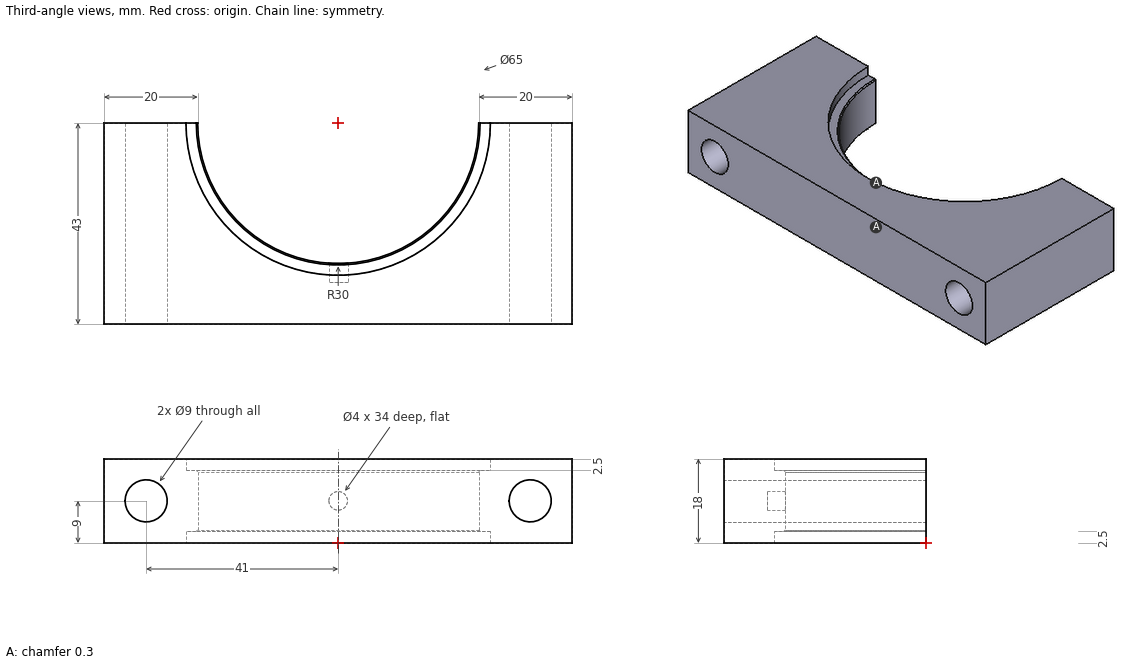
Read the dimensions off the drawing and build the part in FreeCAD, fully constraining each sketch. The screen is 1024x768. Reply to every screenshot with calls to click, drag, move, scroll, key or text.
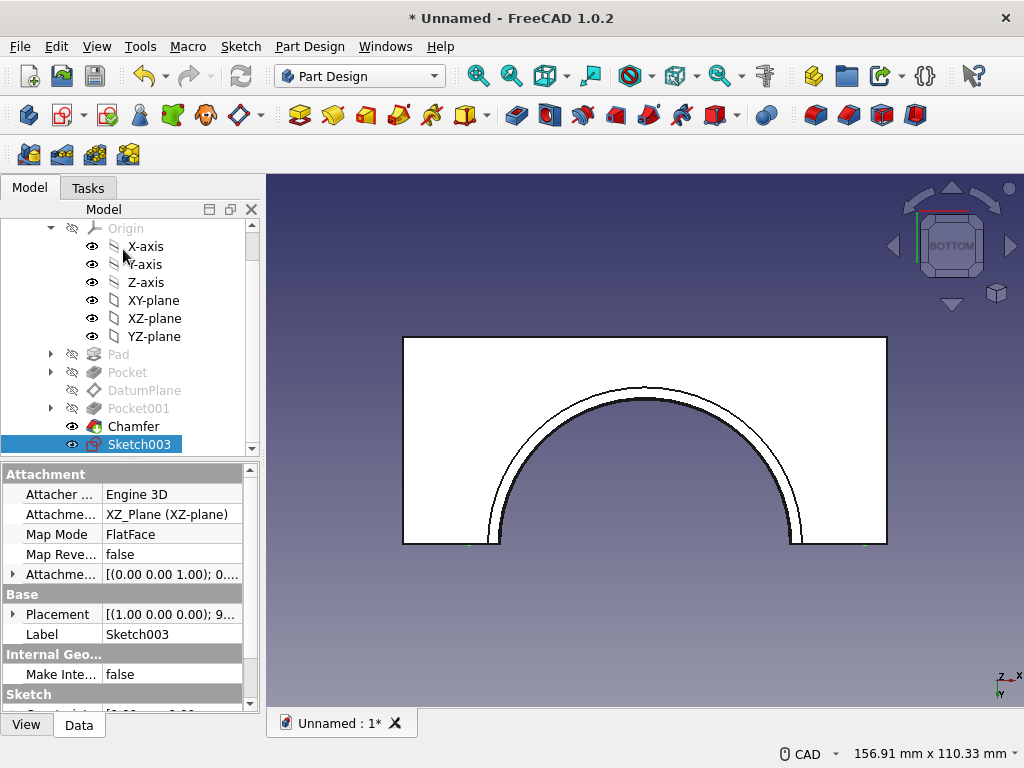
click(550, 116)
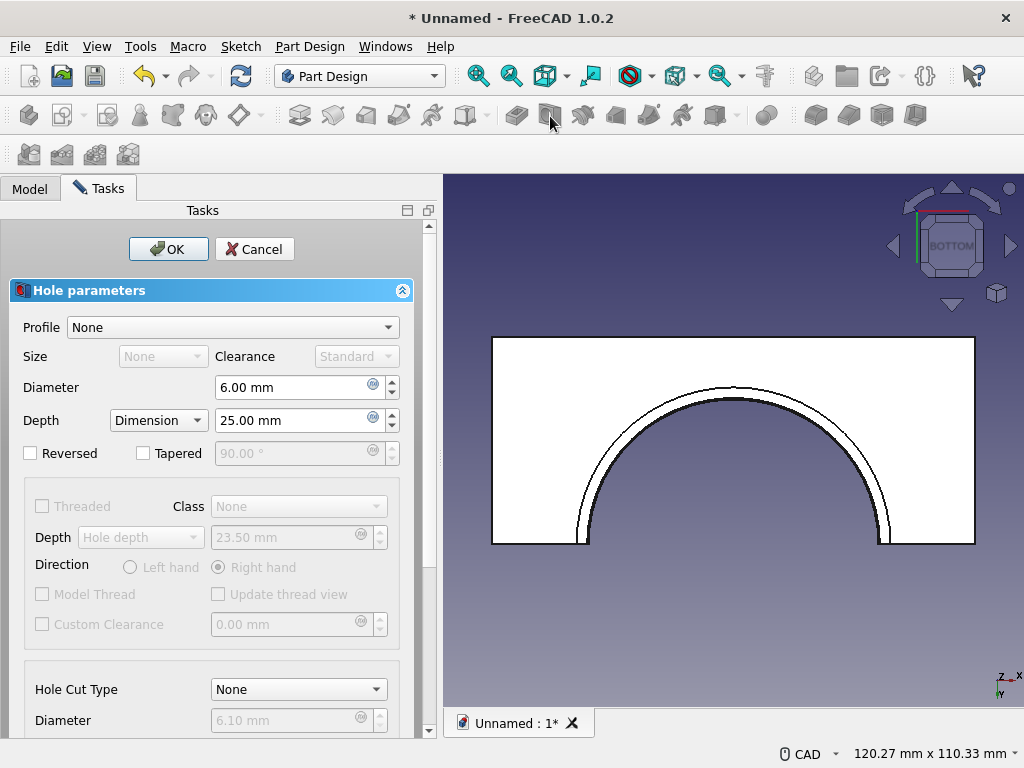
triple_click(300, 388)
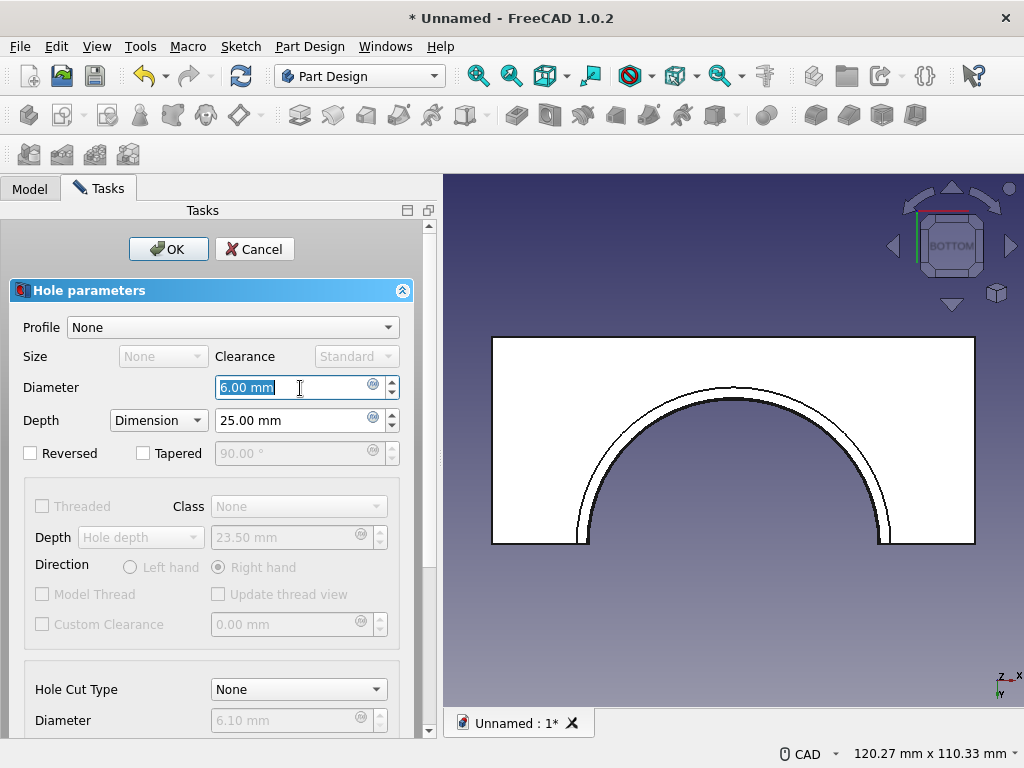
text(9)
key(Tab)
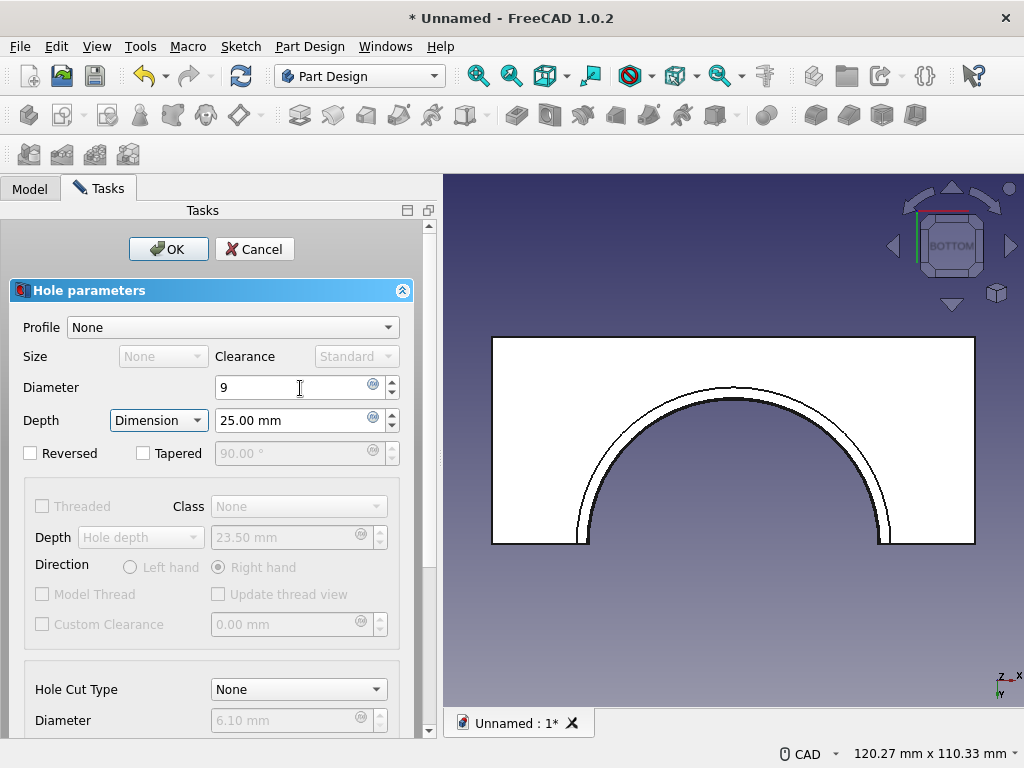
click(160, 420)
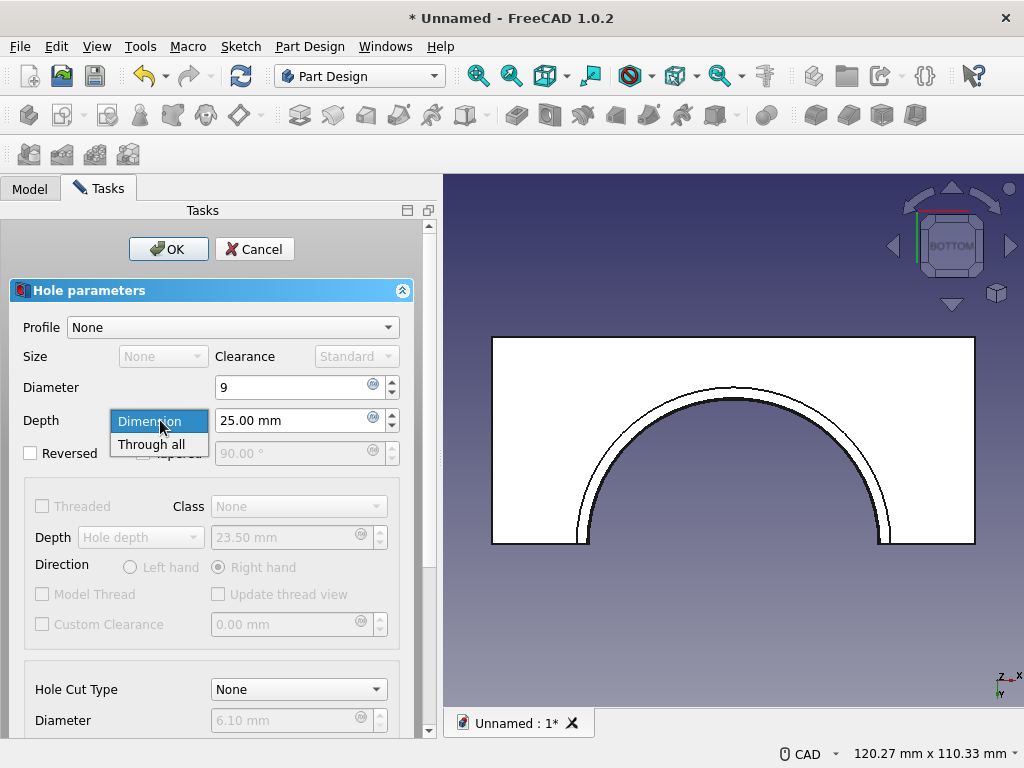
click(158, 444)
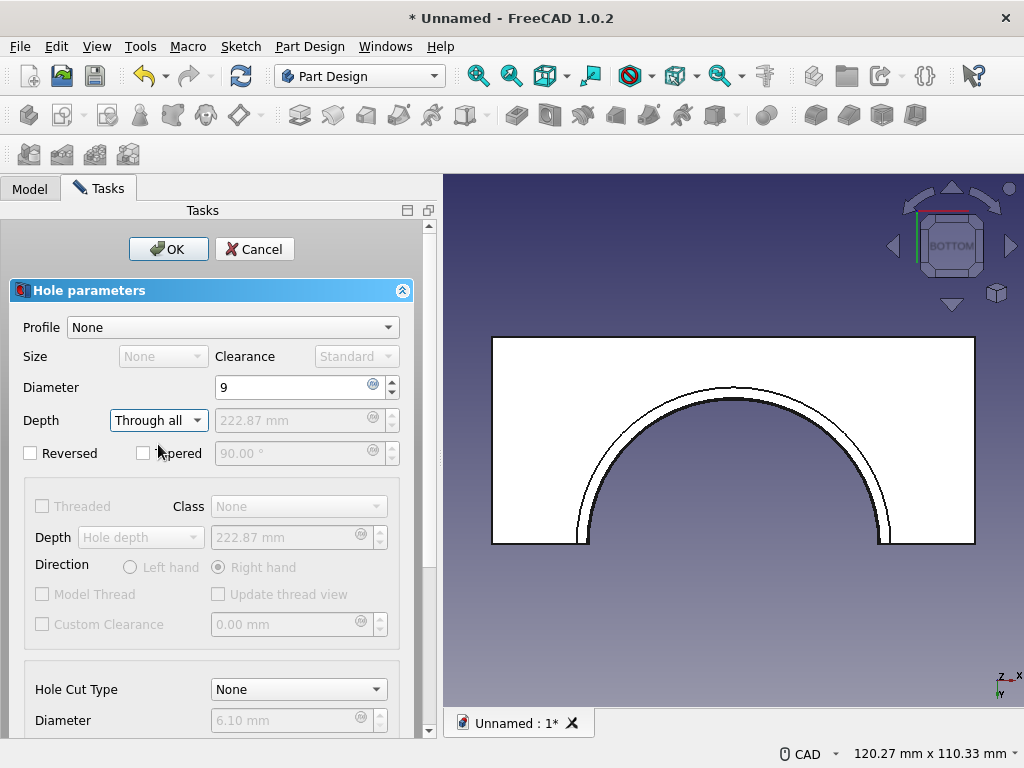
click(31, 453)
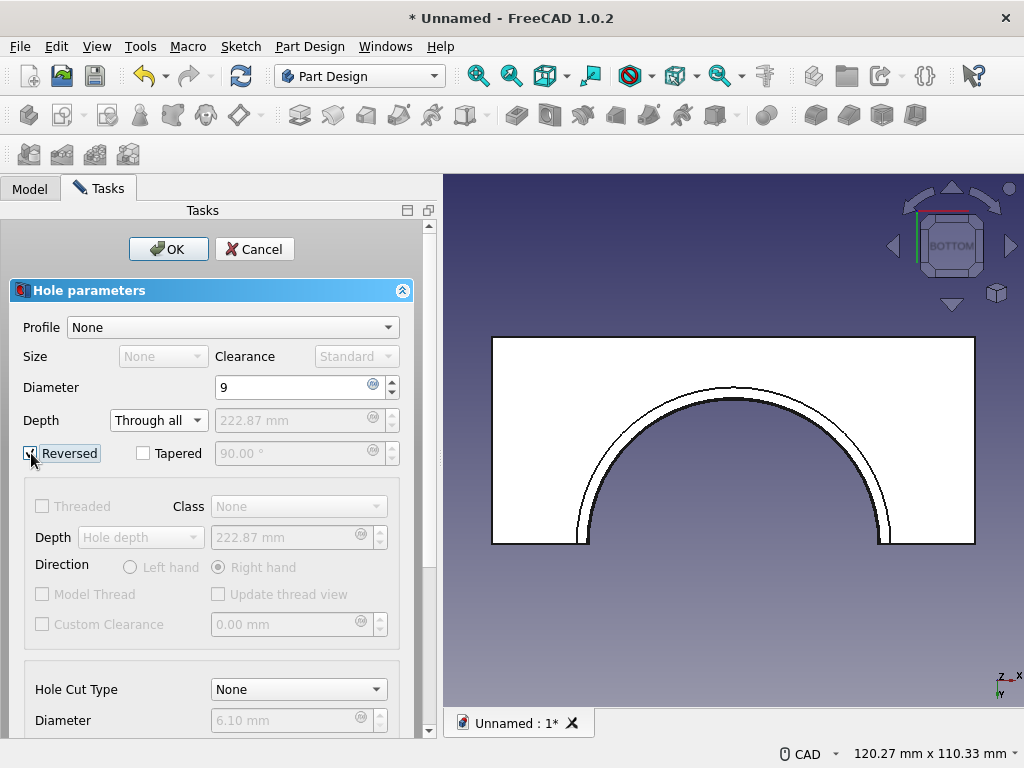
click(169, 249)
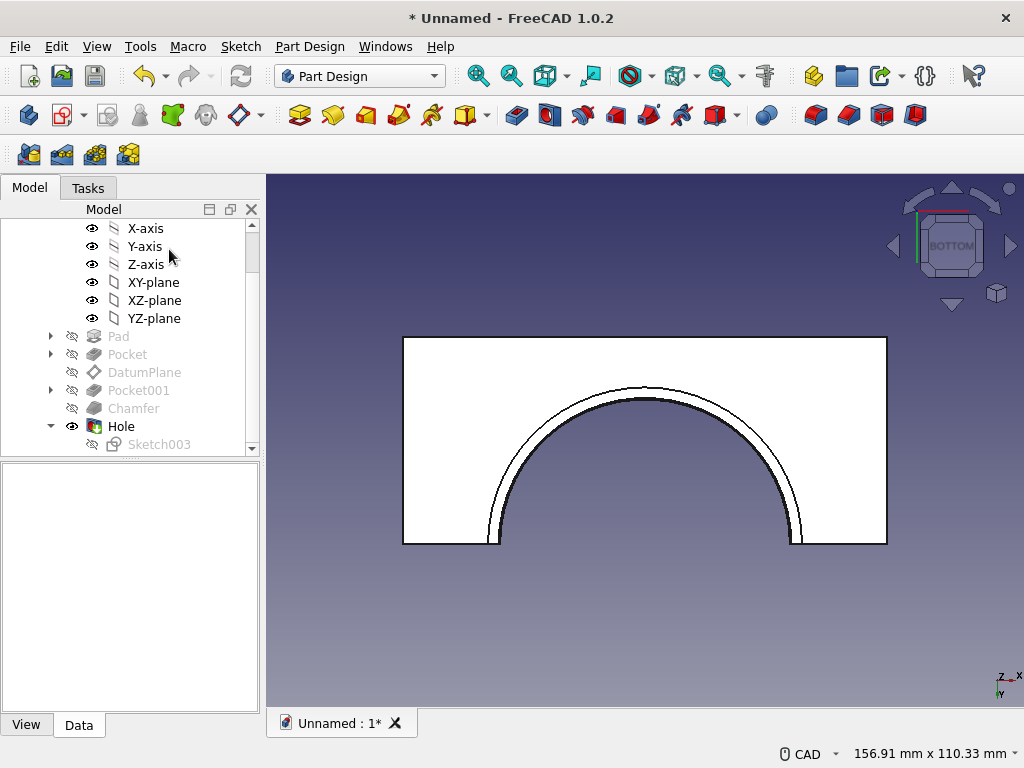
click(62, 116)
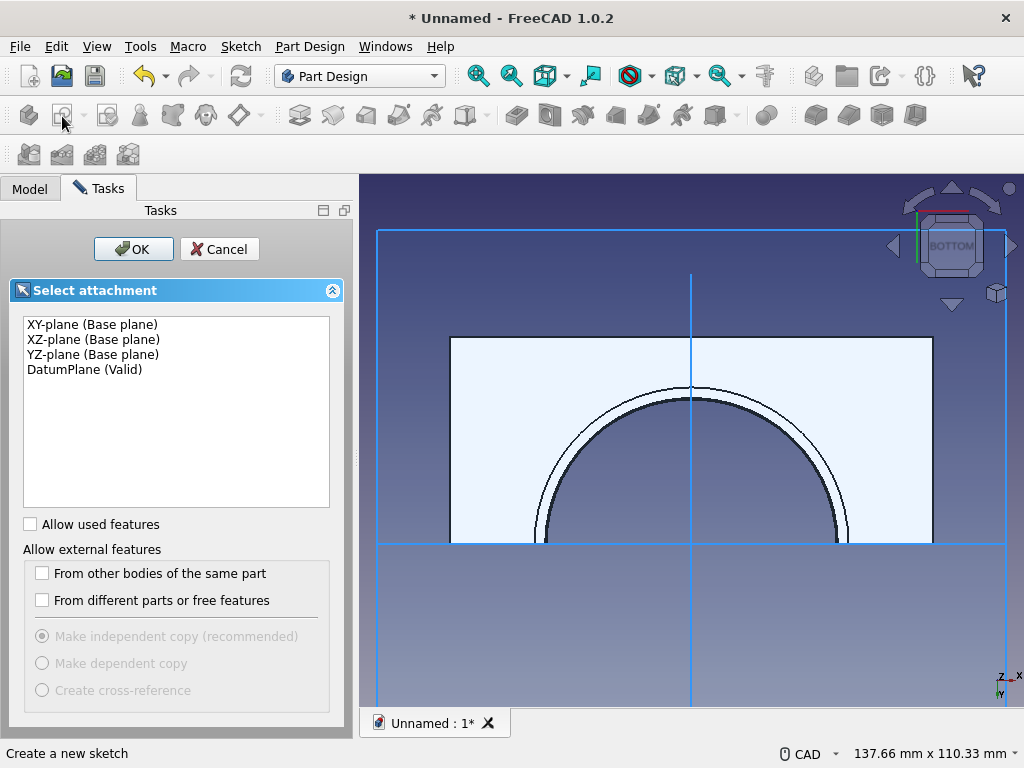
click(84, 340)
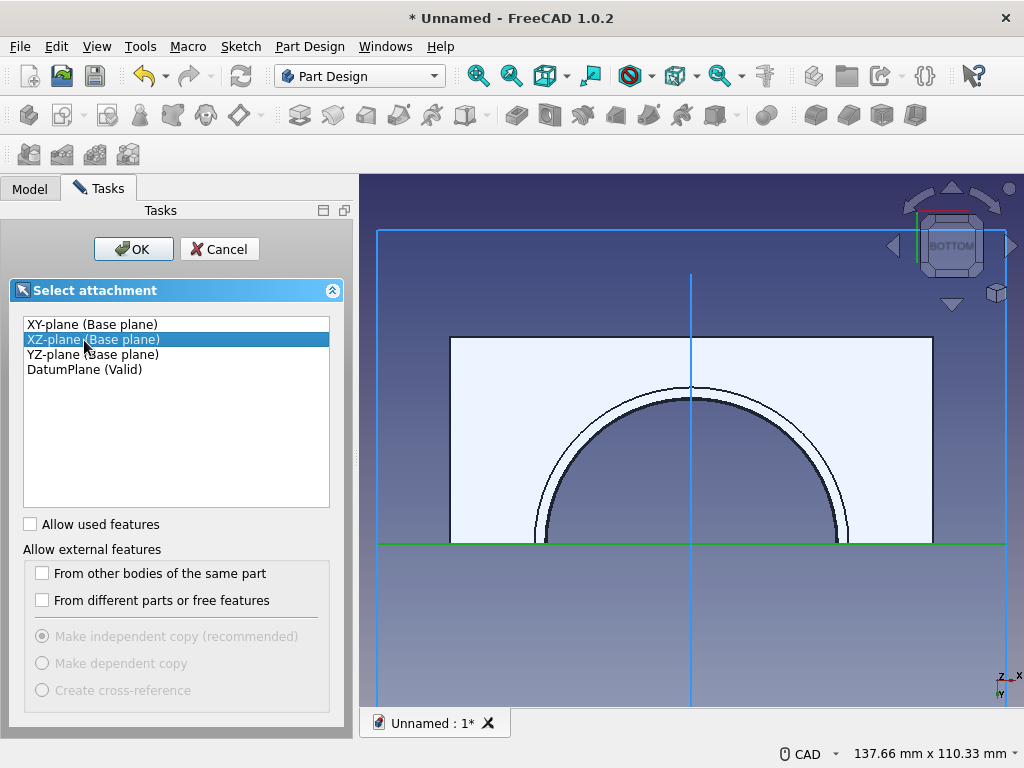
click(134, 249)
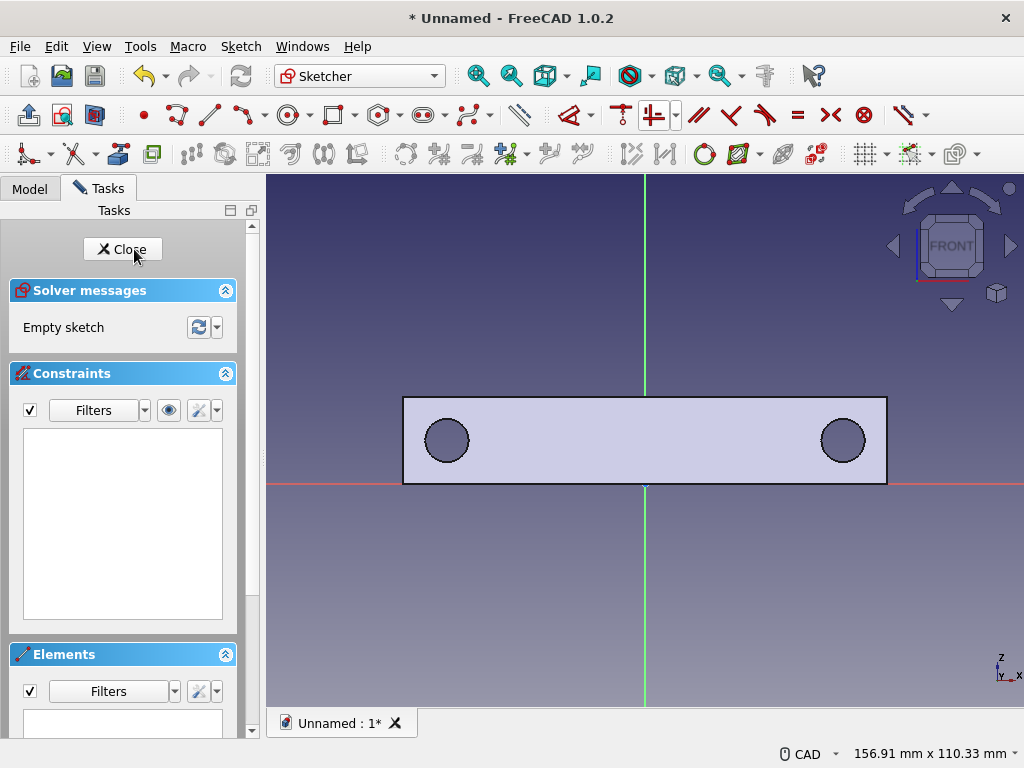
click(95, 116)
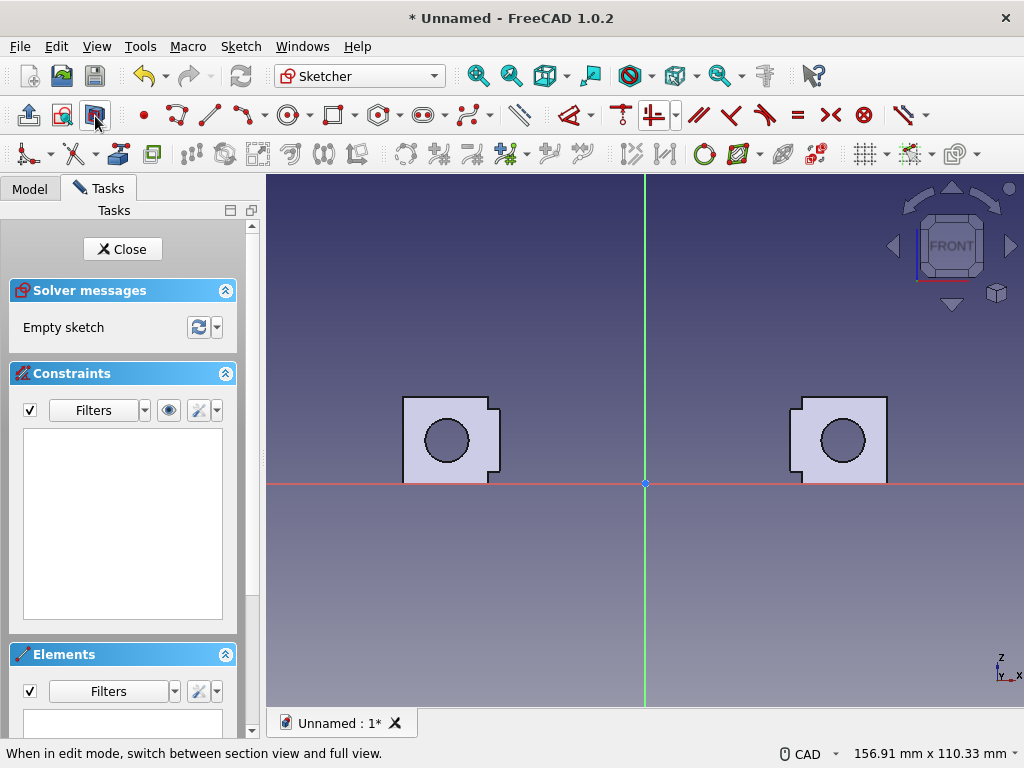
scroll(649, 440, up, 14)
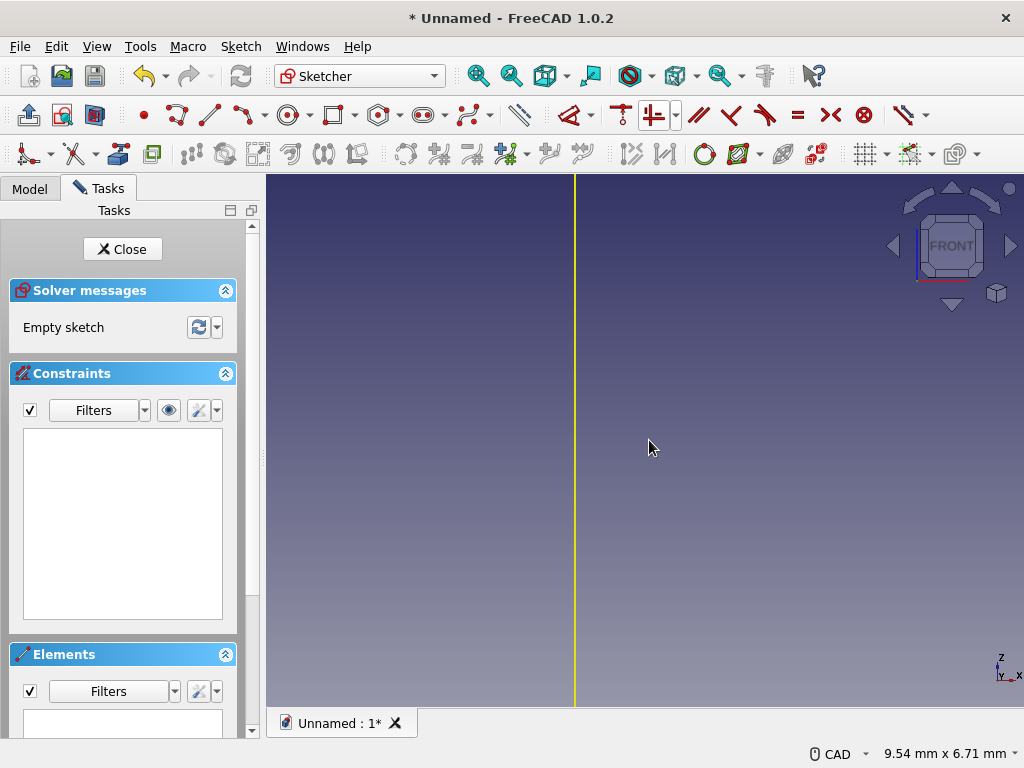
click(288, 116)